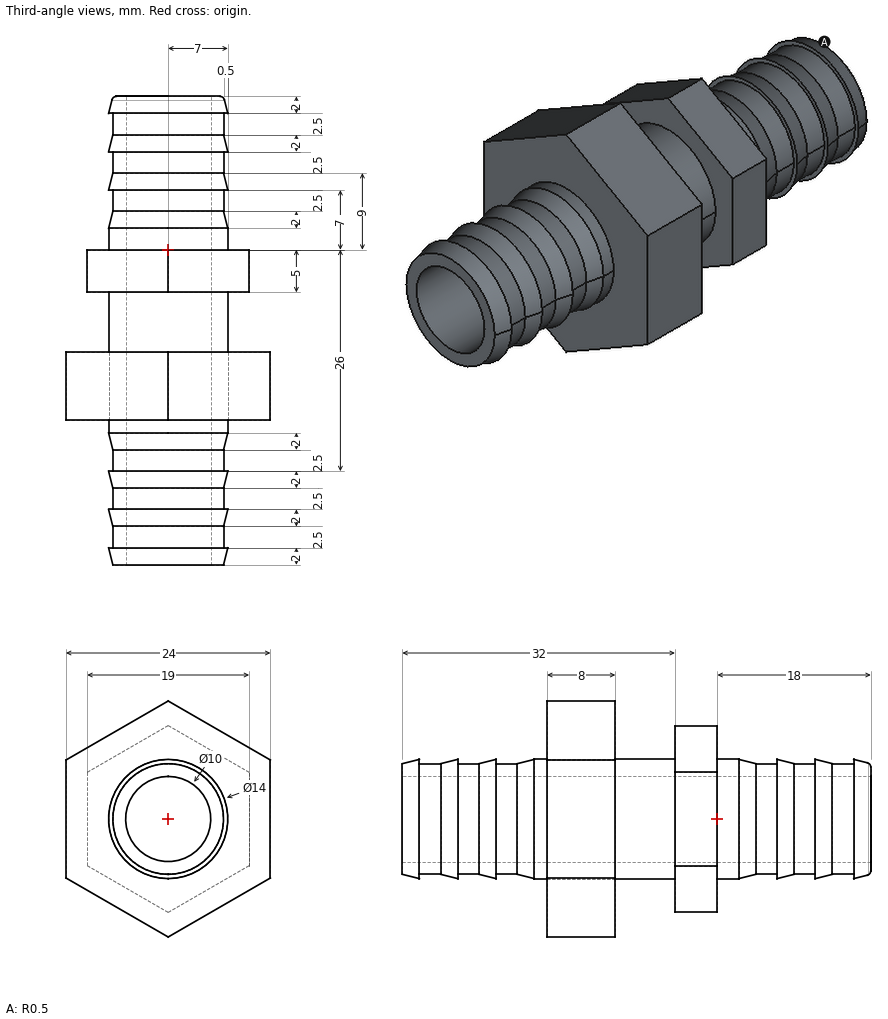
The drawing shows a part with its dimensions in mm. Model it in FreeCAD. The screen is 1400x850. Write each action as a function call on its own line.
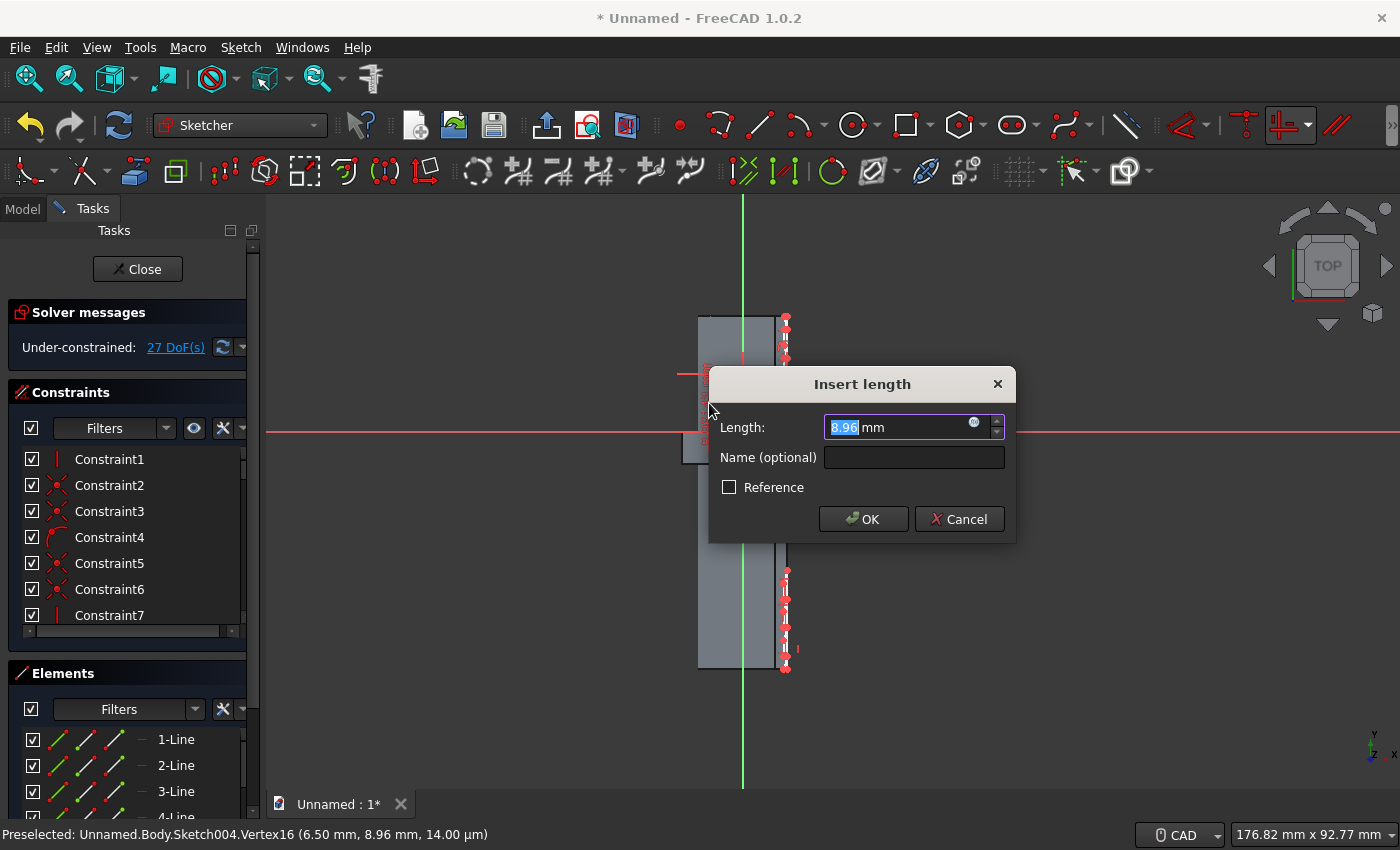
text(9)
key(Return)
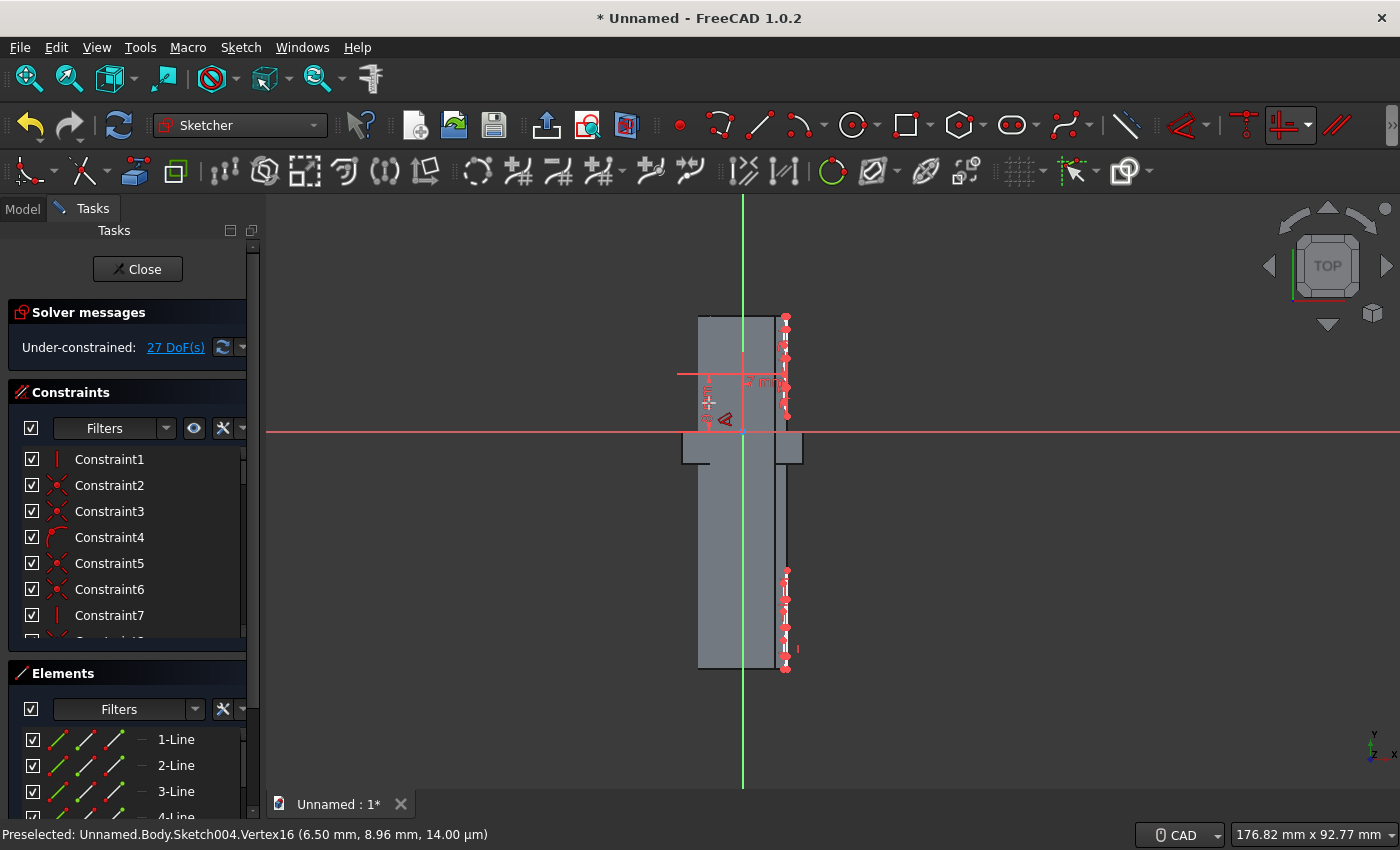
scroll(787, 388, up, 7)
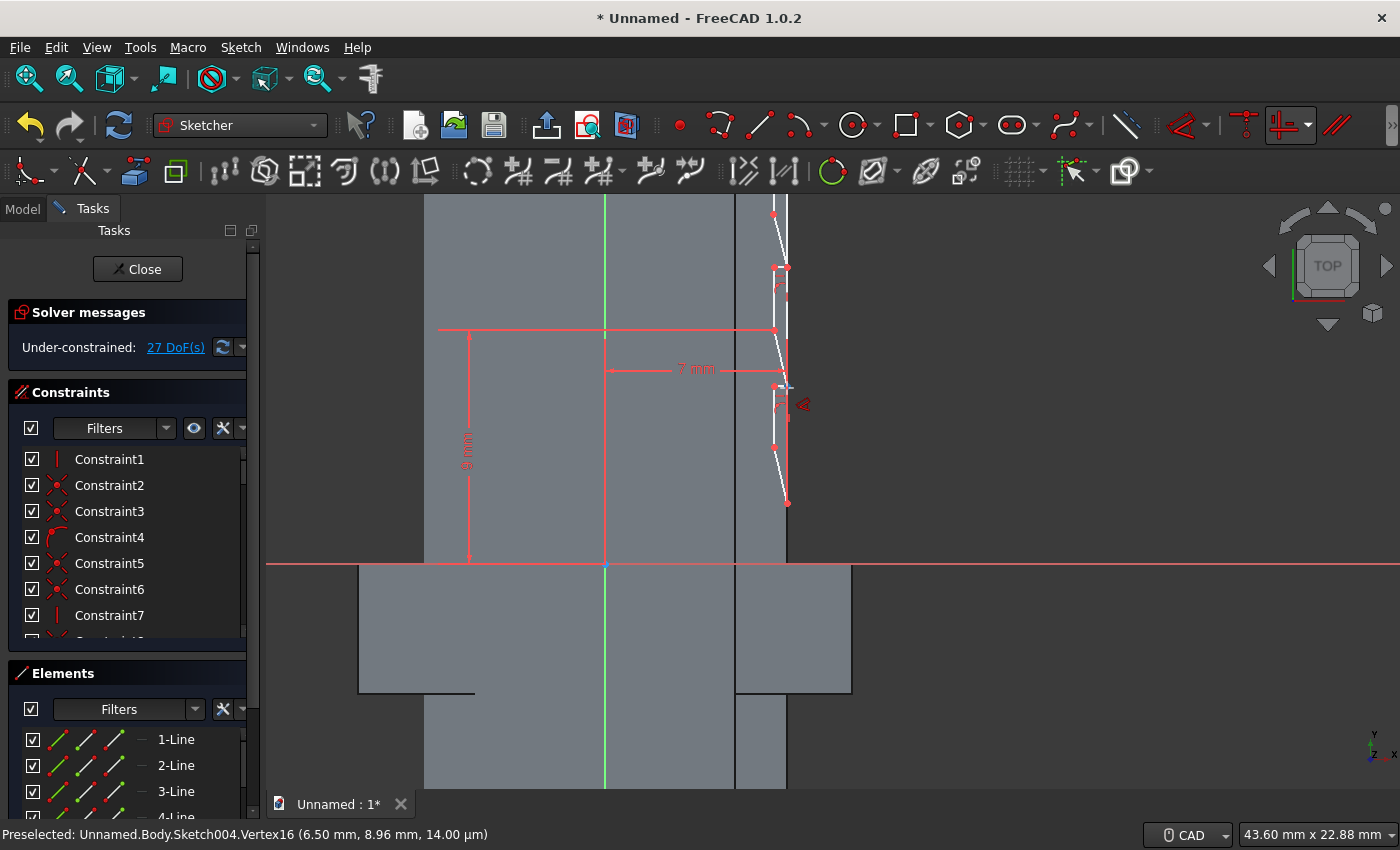
click(787, 386)
click(571, 475)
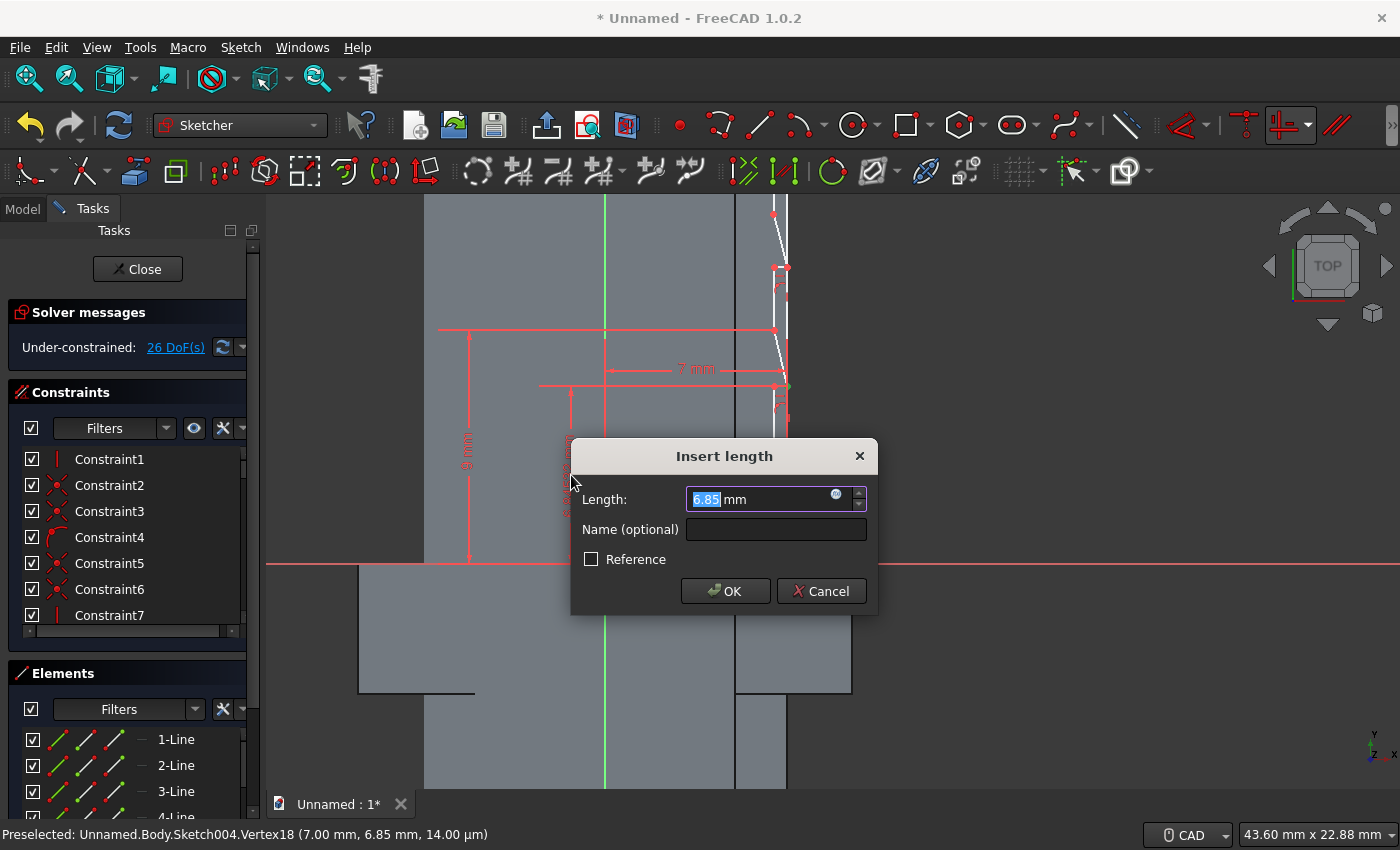
text(7)
key(Return)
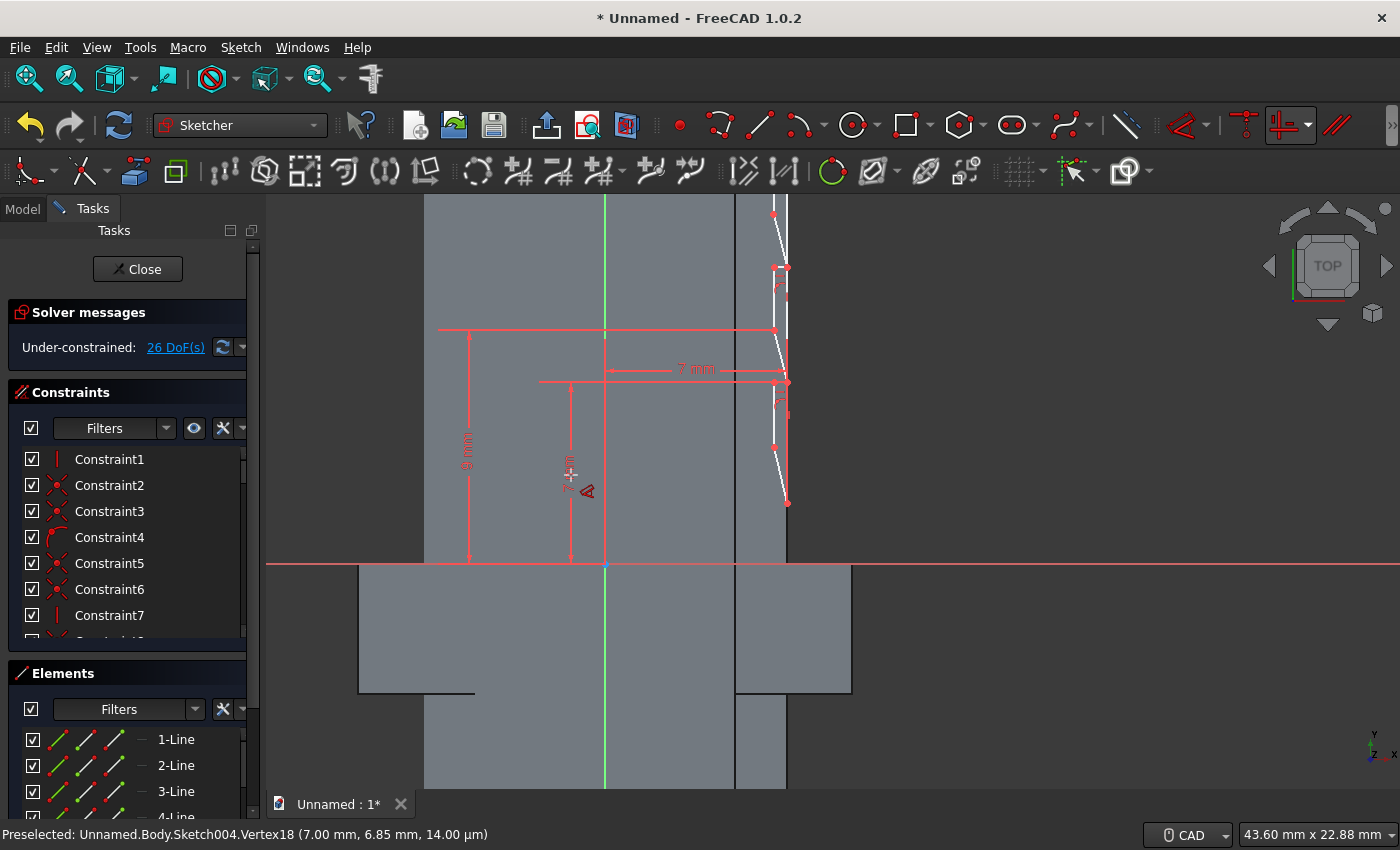
scroll(787, 387, down, 7)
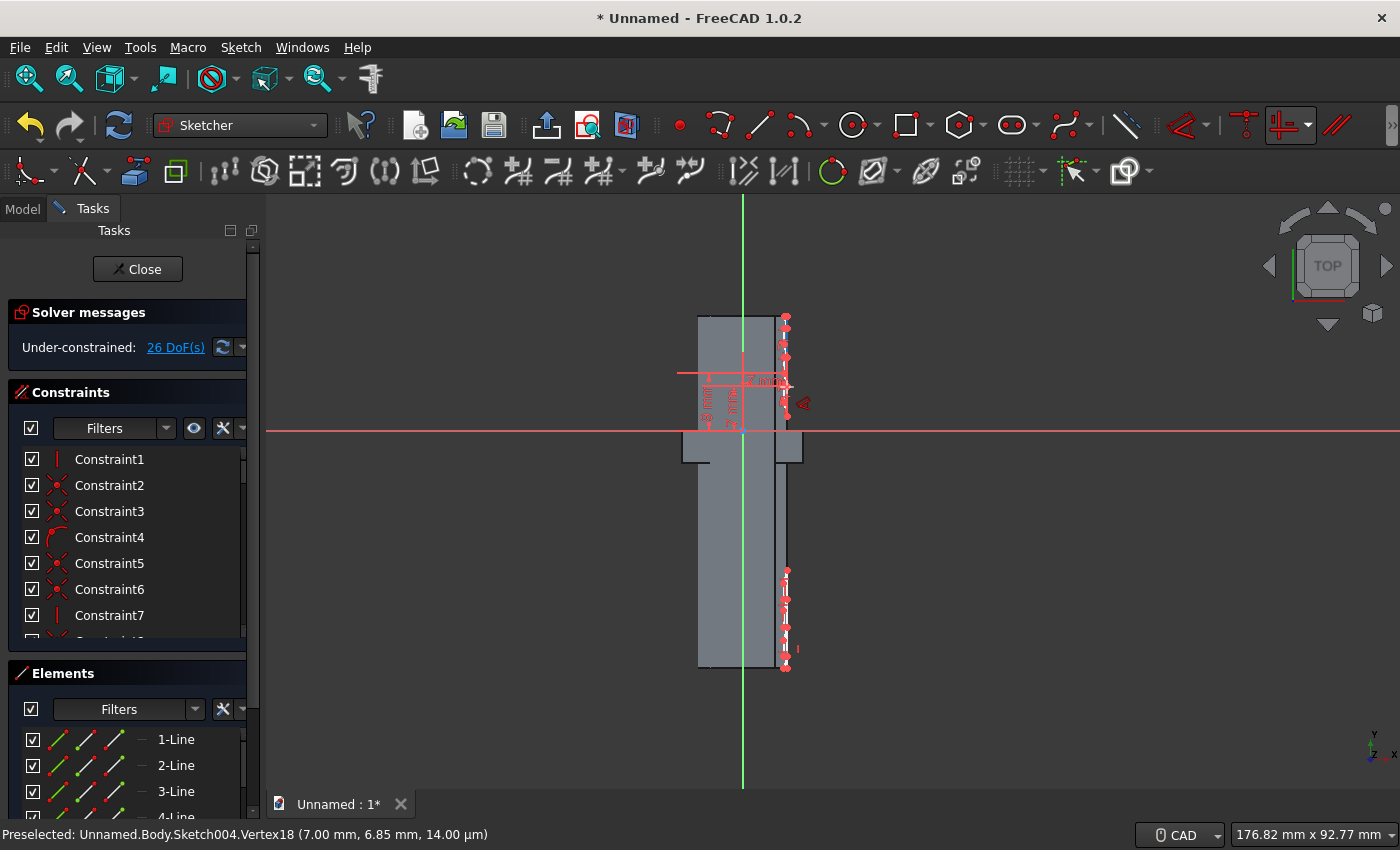
click(787, 570)
click(765, 604)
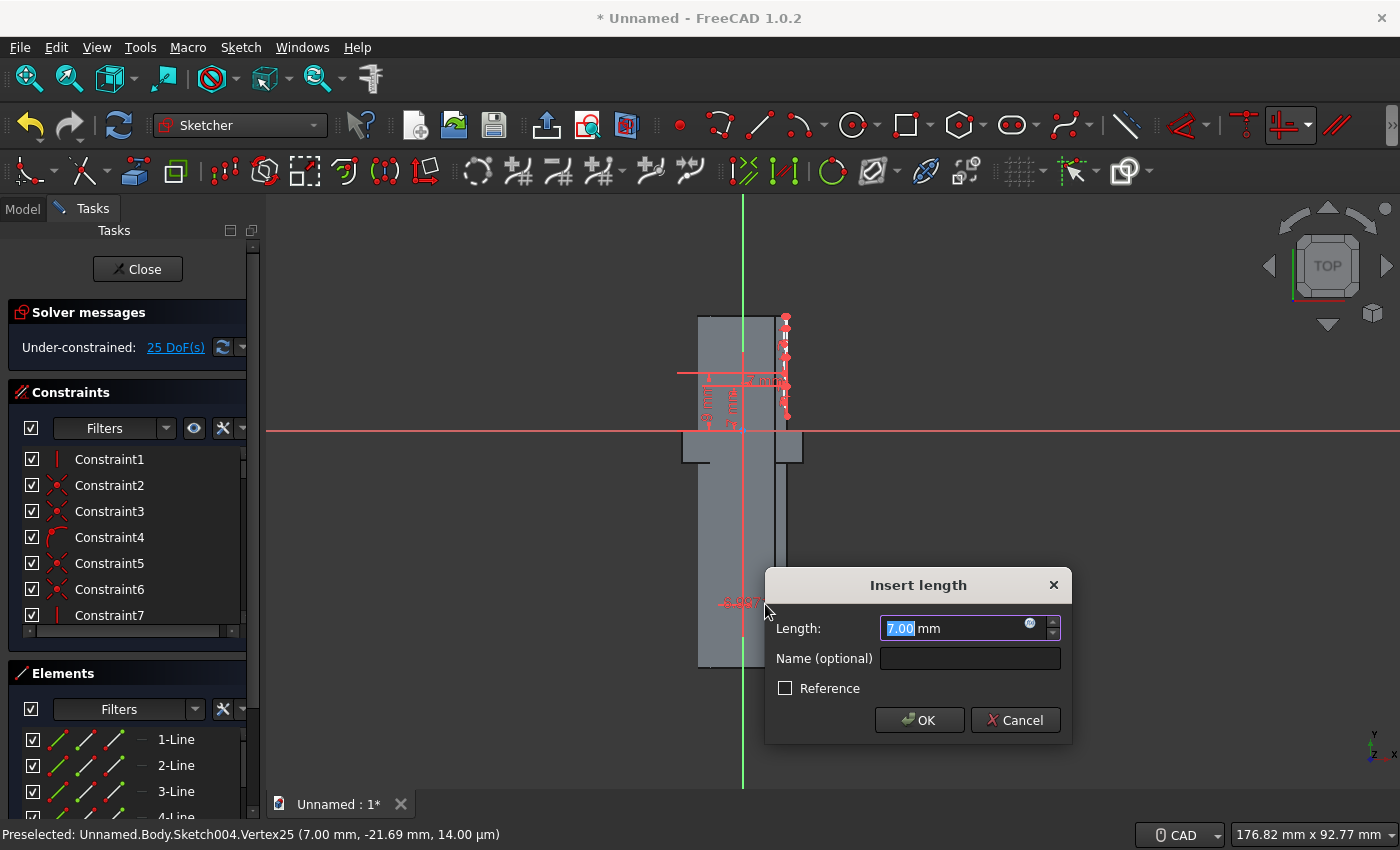
text(7)
key(Return)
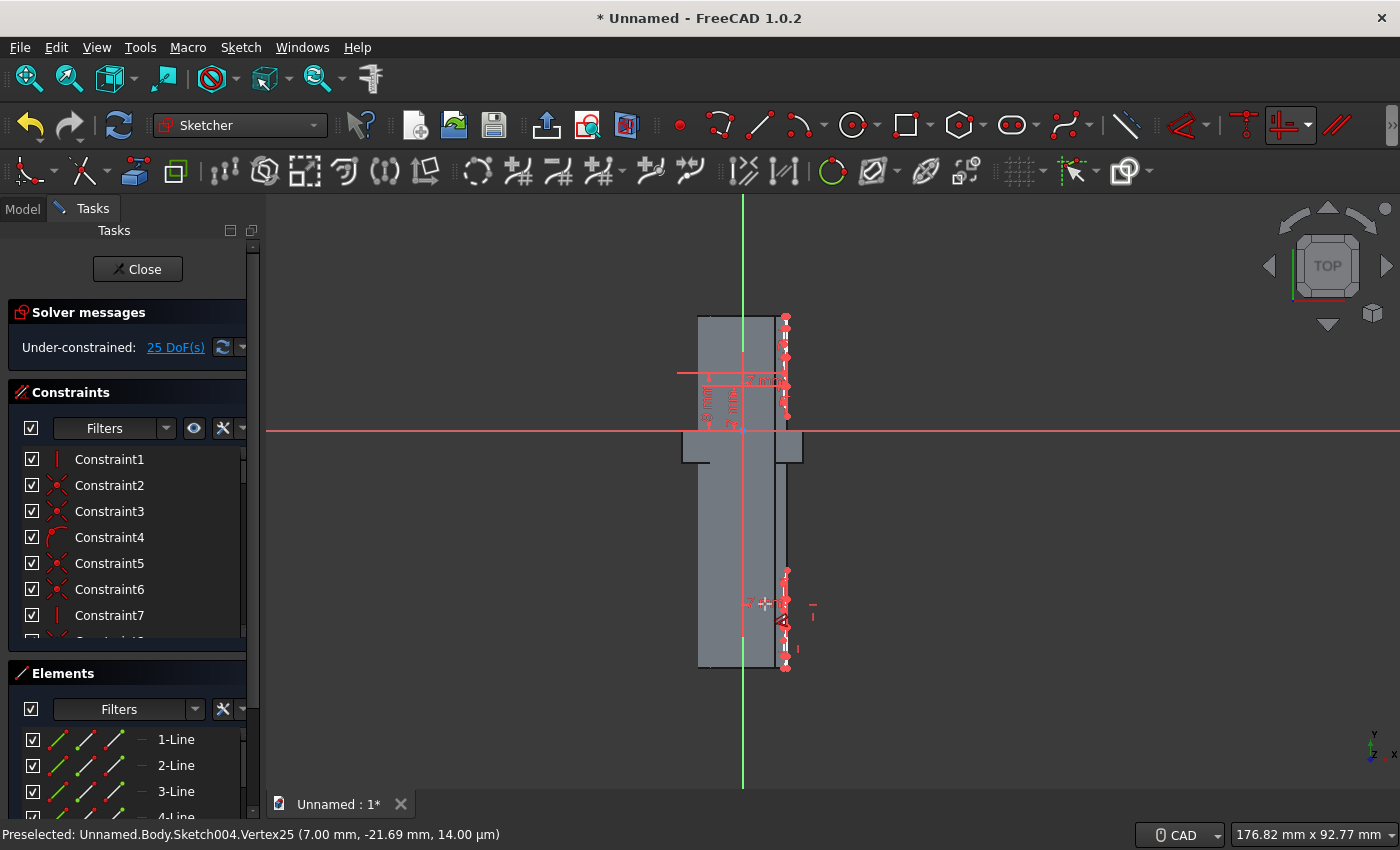
scroll(787, 599, up, 7)